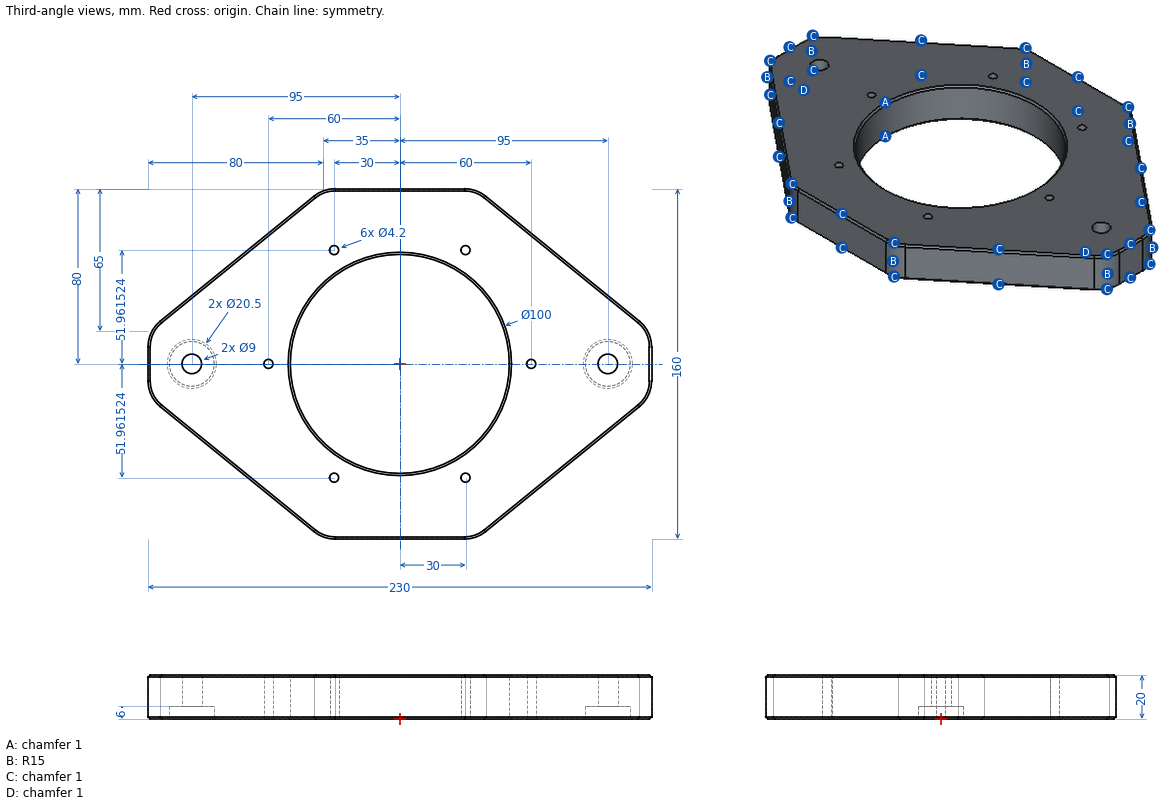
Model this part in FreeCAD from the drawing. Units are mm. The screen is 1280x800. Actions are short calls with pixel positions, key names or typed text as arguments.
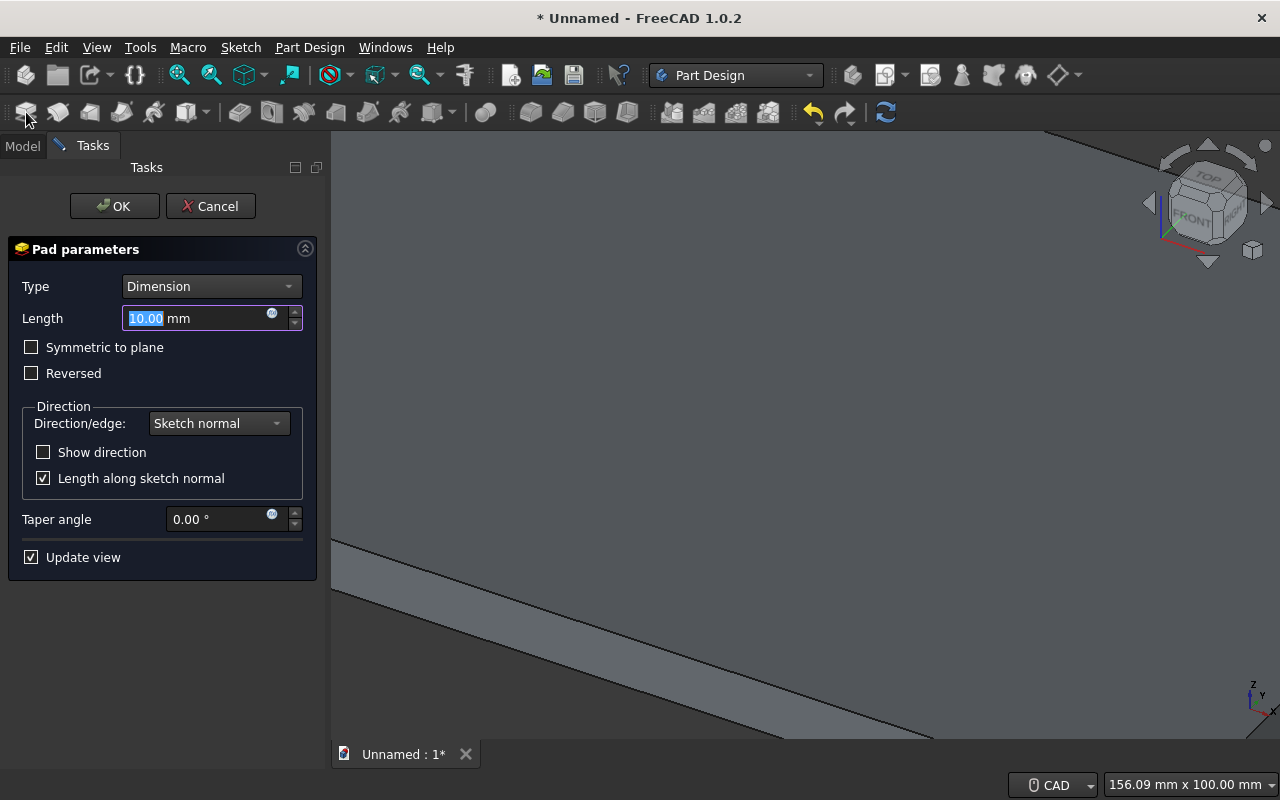
text(20)
key(Tab)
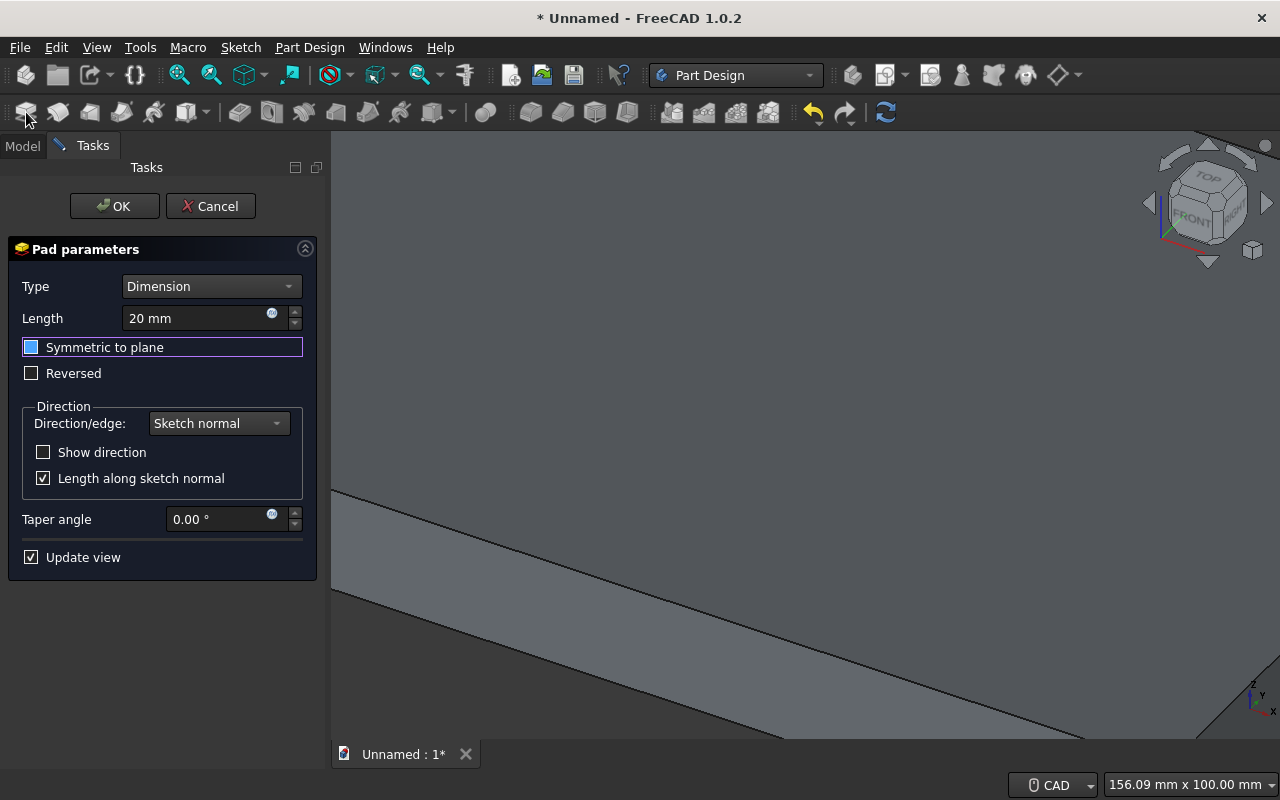
click(115, 206)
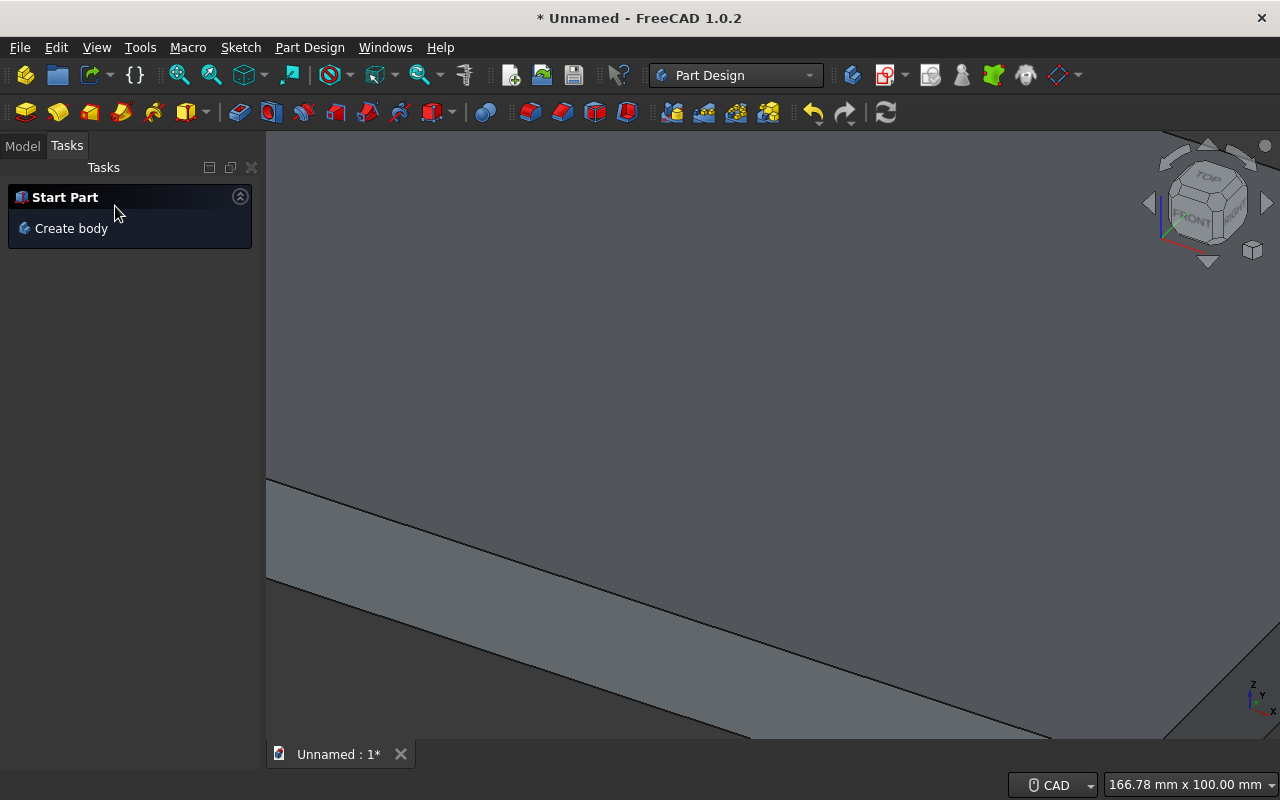
click(180, 76)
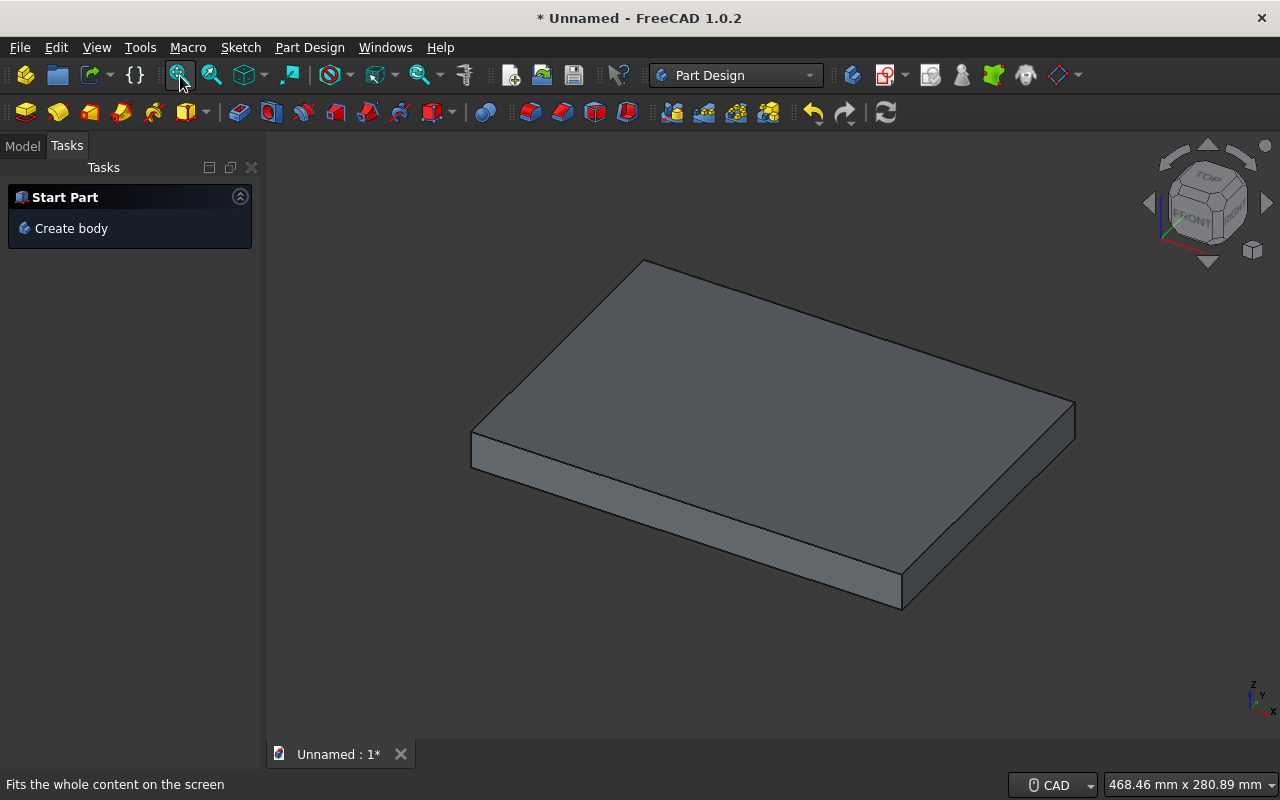
click(835, 437)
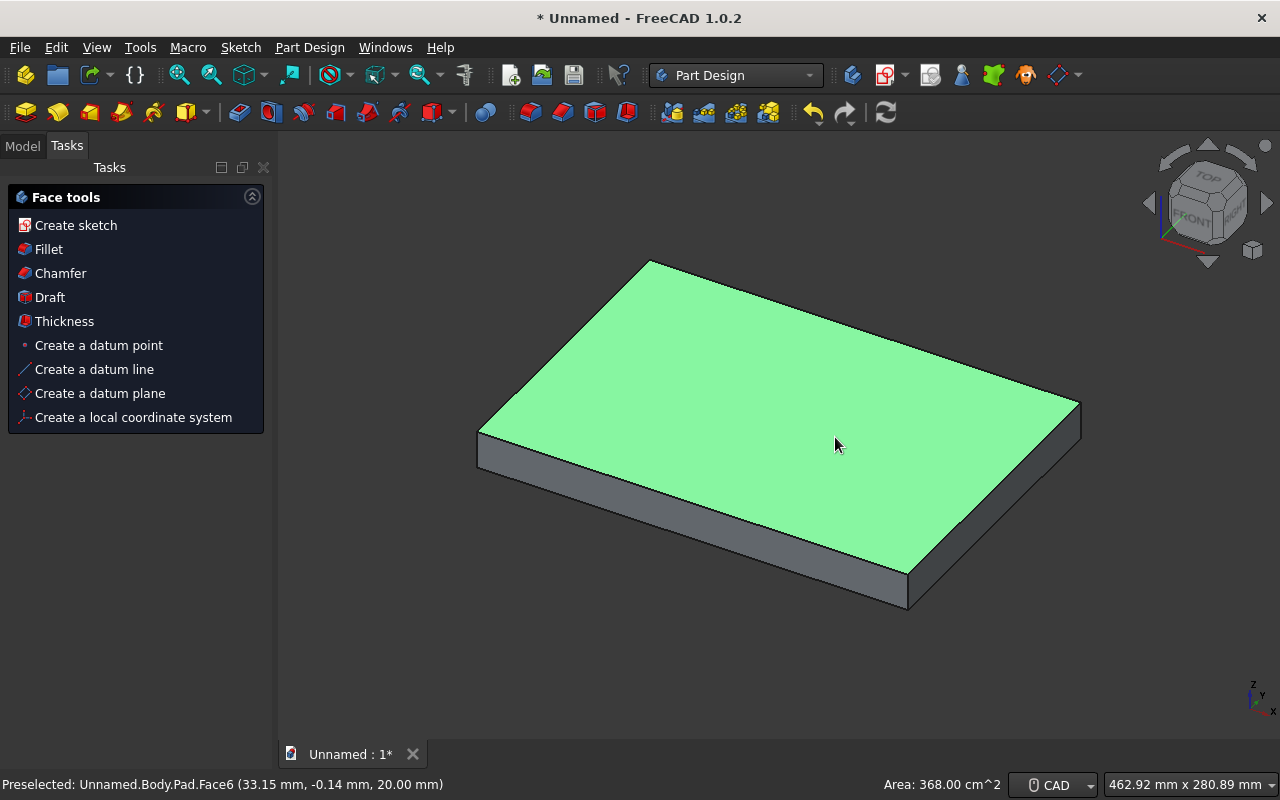
click(886, 76)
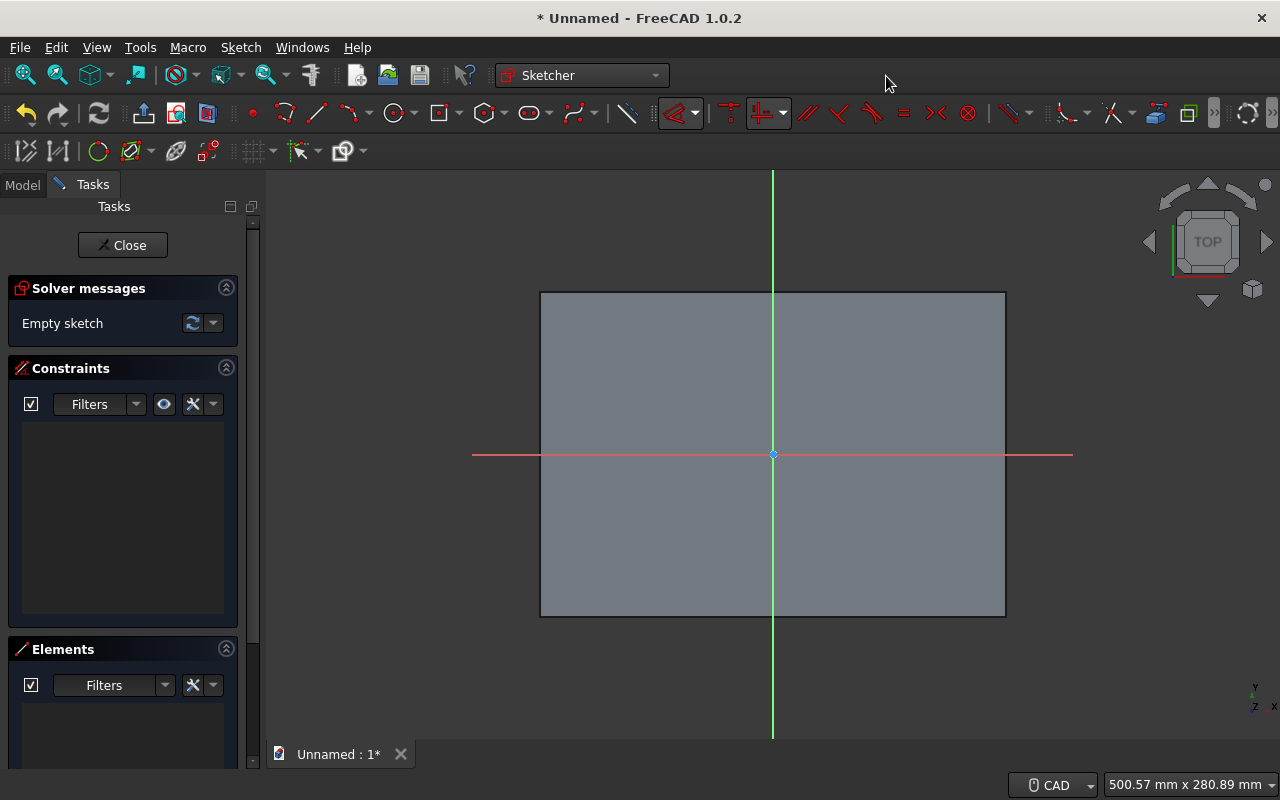
scroll(856, 454, up, 3)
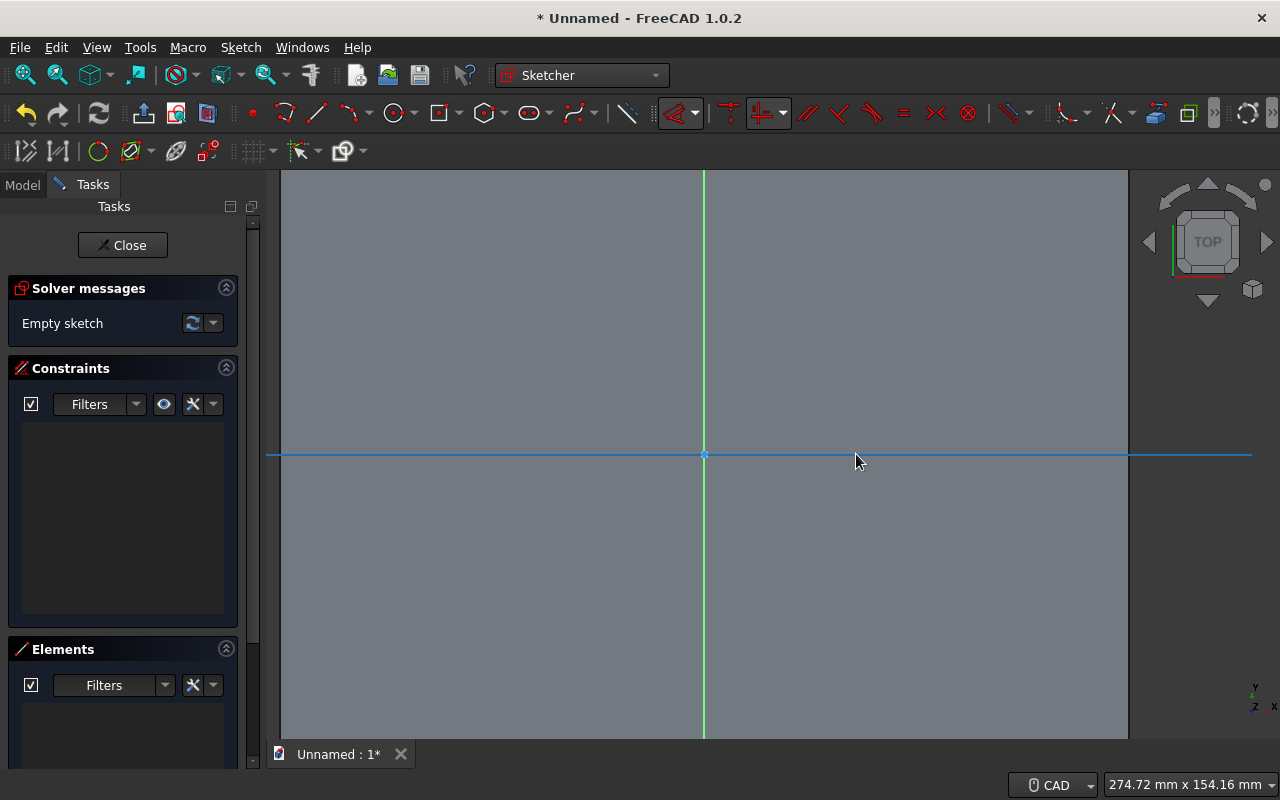
click(394, 114)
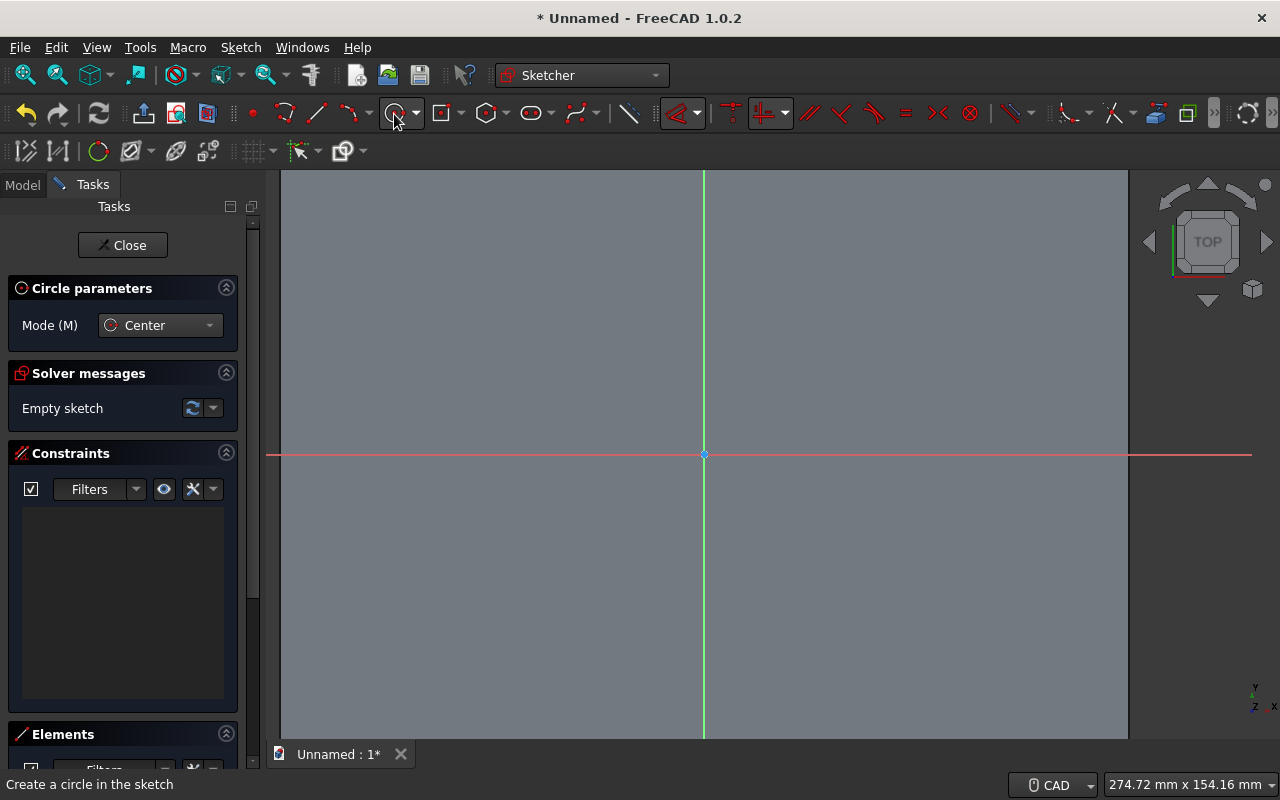
click(704, 454)
move(835, 324)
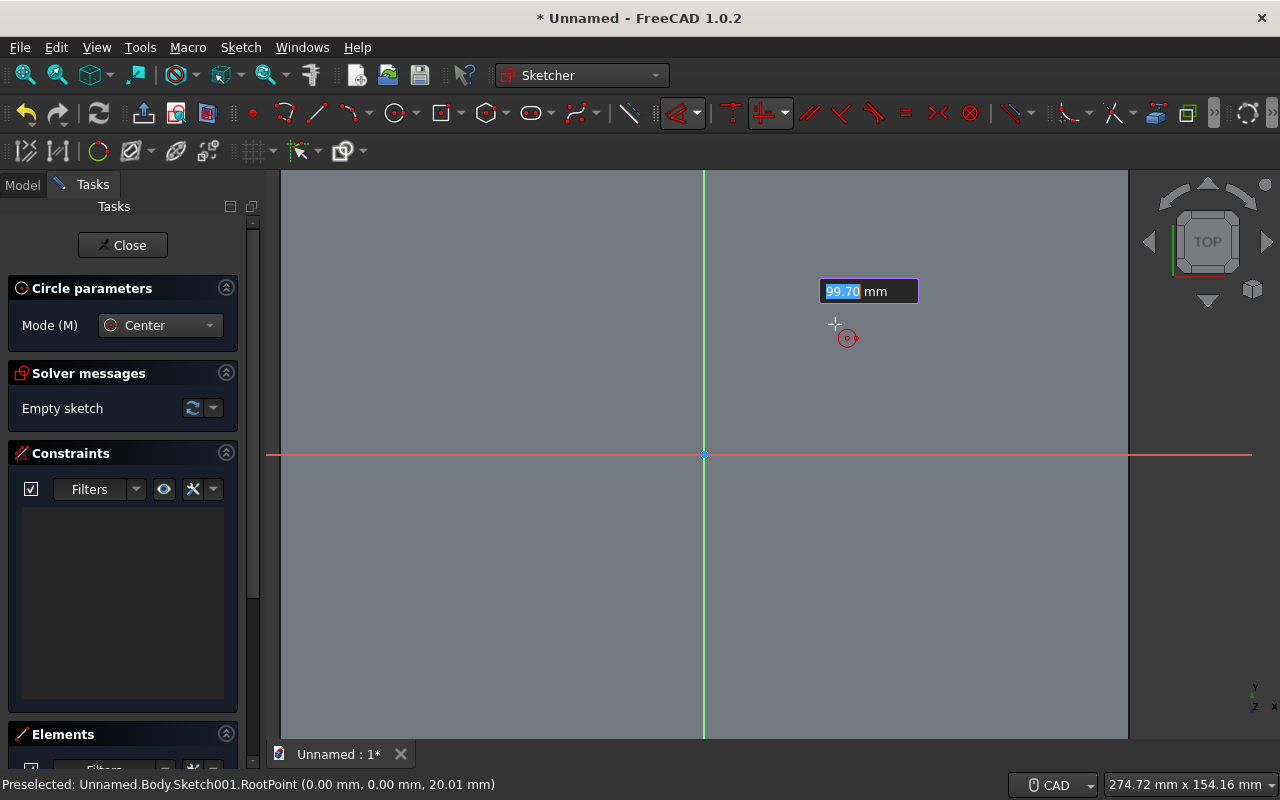
text(100)
key(Return)
key(Escape)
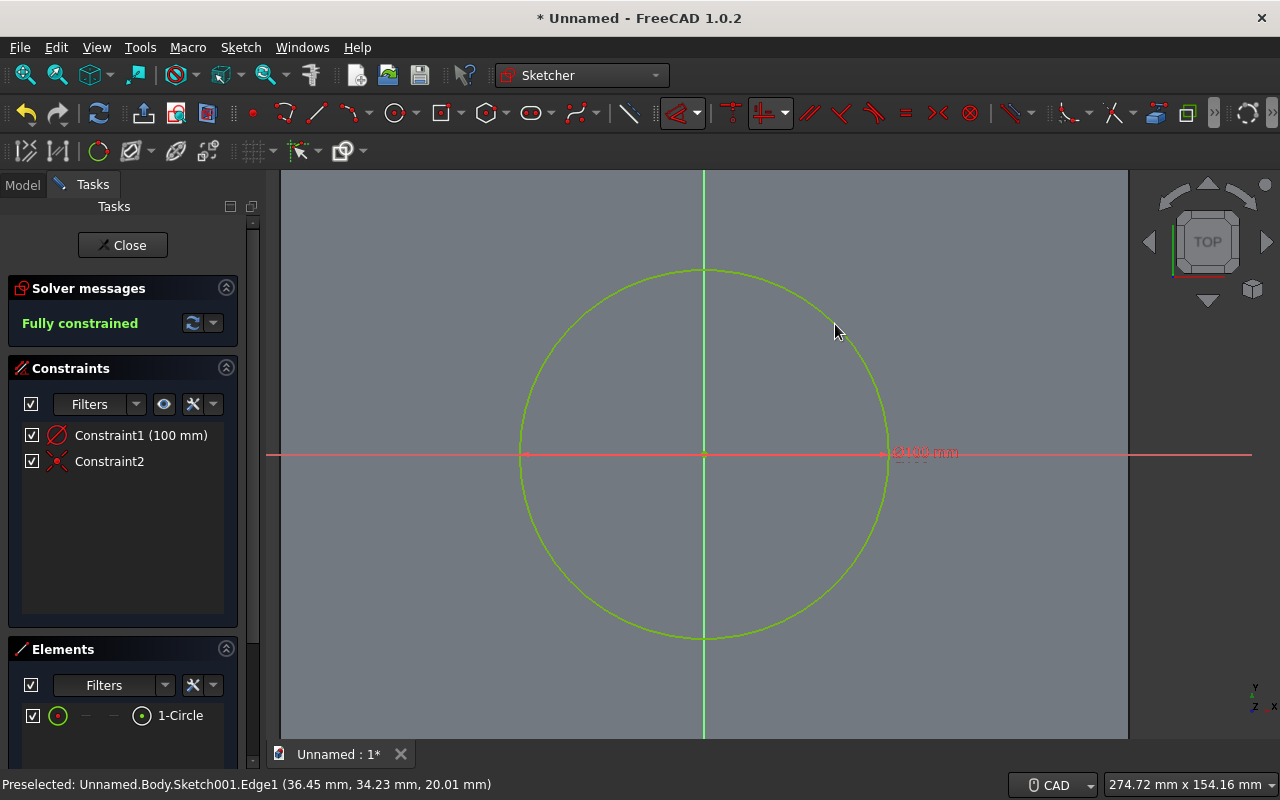
click(123, 245)